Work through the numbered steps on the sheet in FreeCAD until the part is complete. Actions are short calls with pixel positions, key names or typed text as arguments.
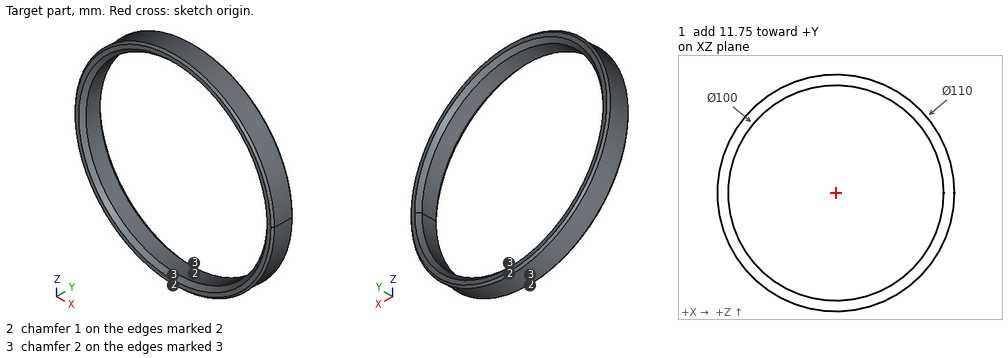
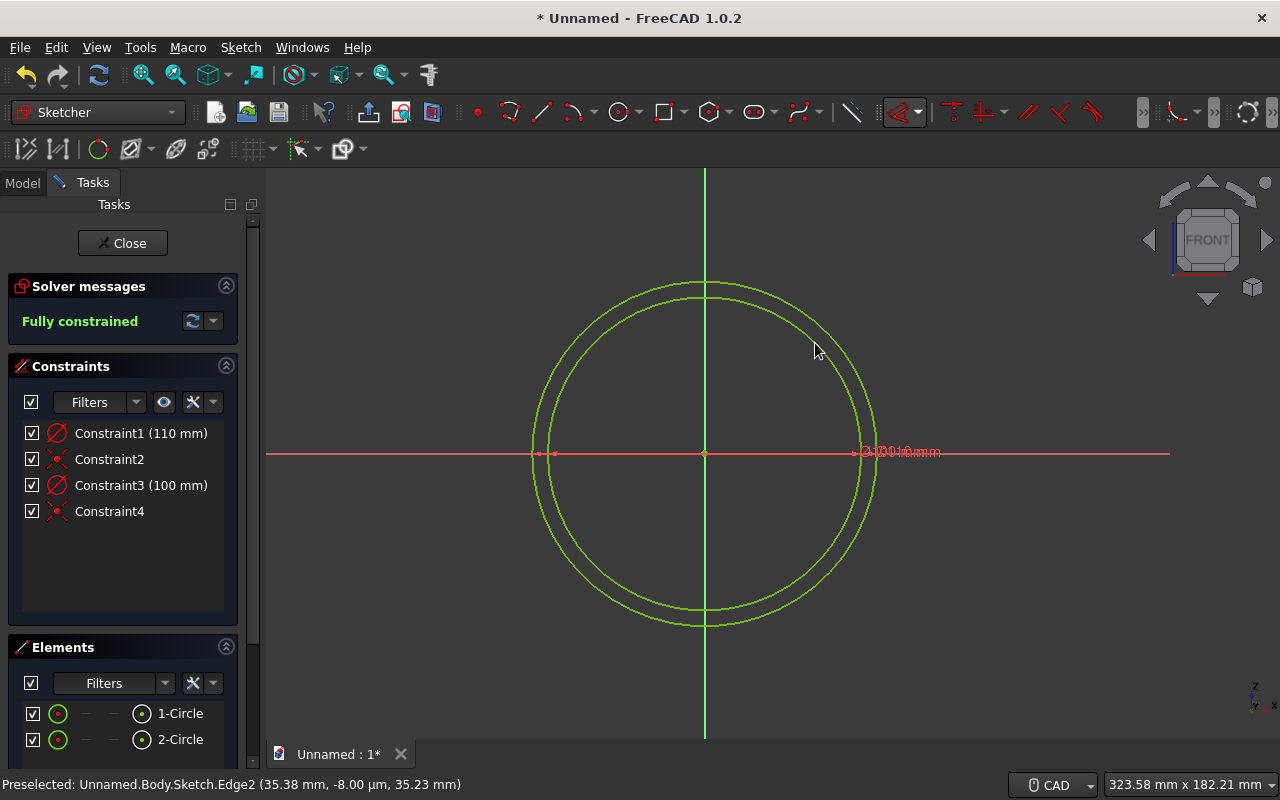
click(123, 243)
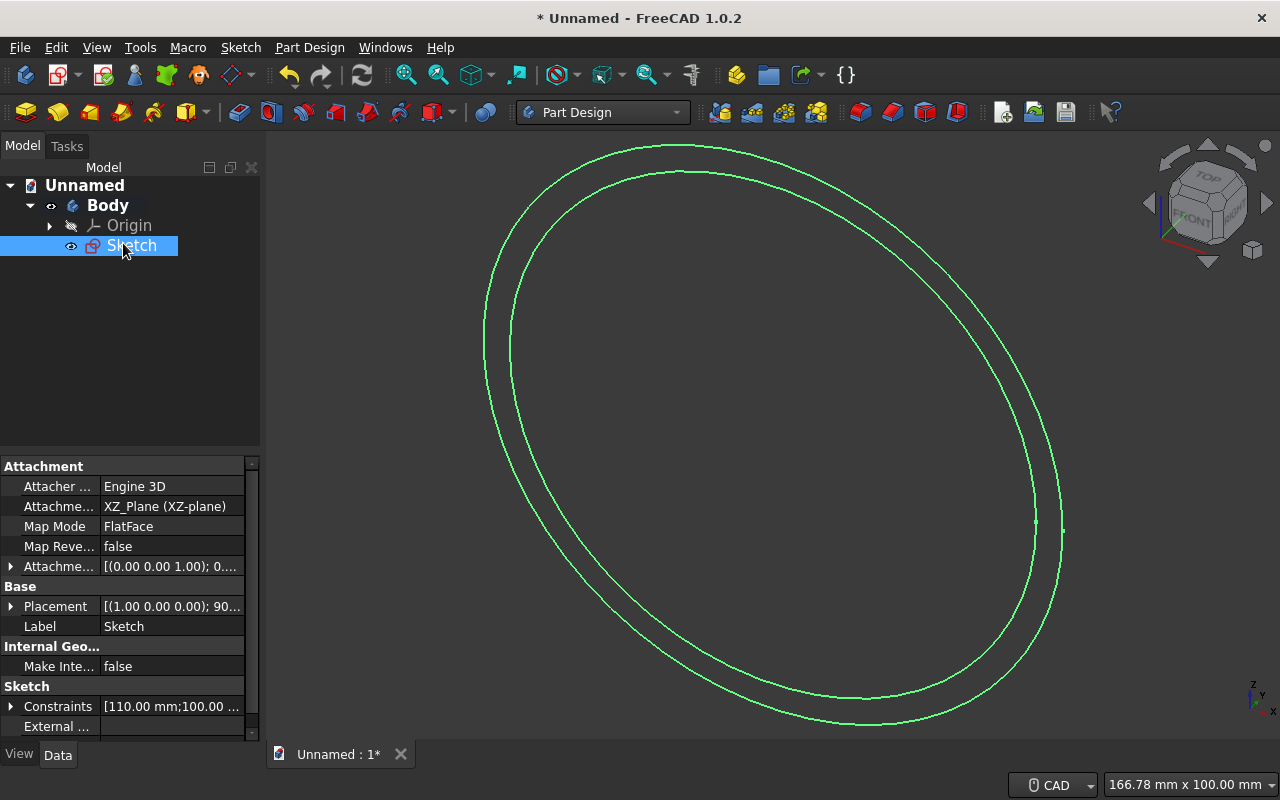
click(26, 112)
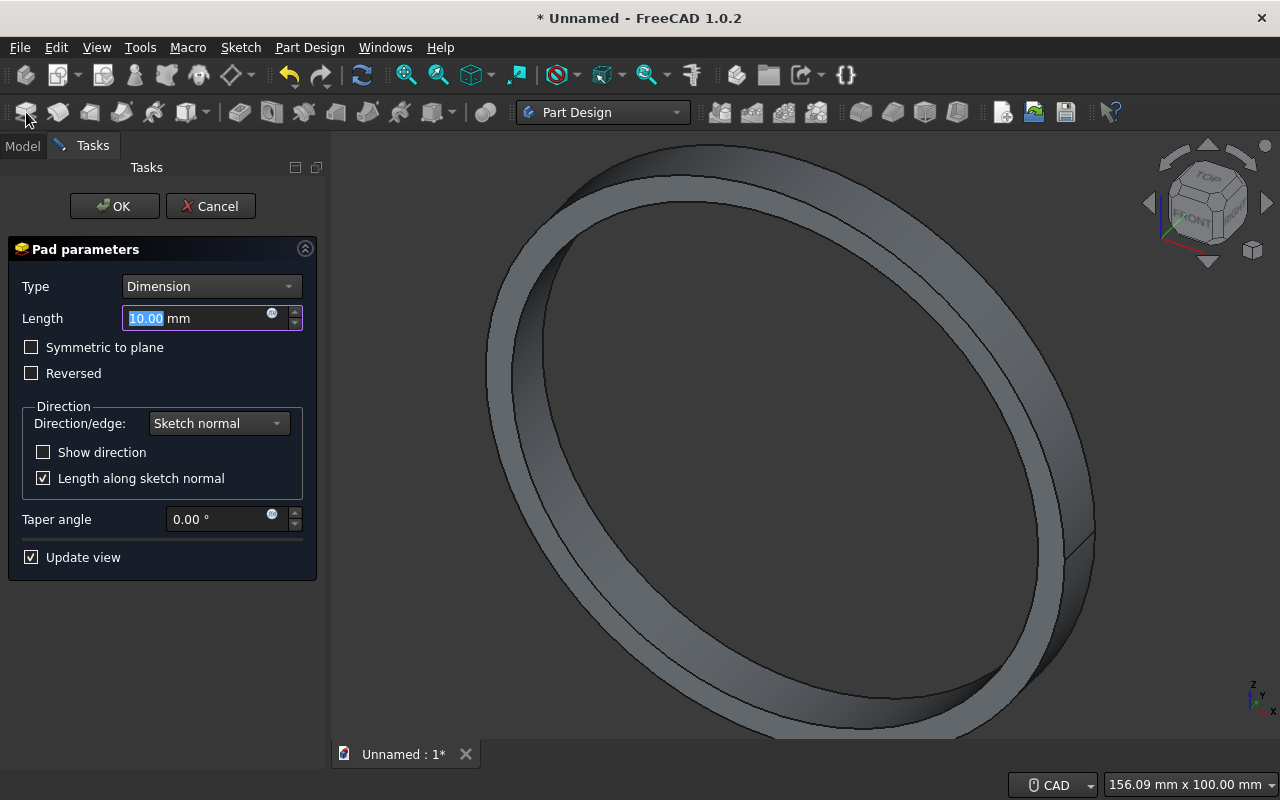
text(11.75)
key(Tab)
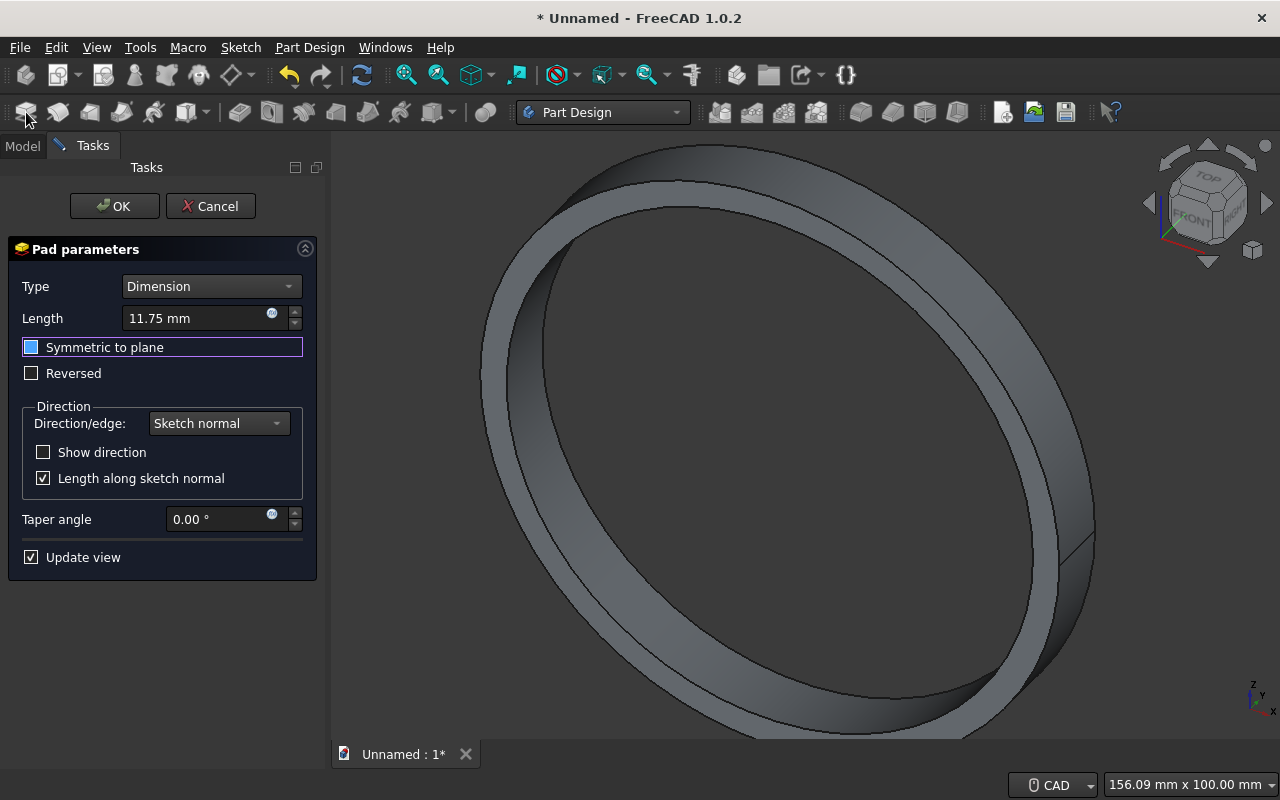
click(30, 373)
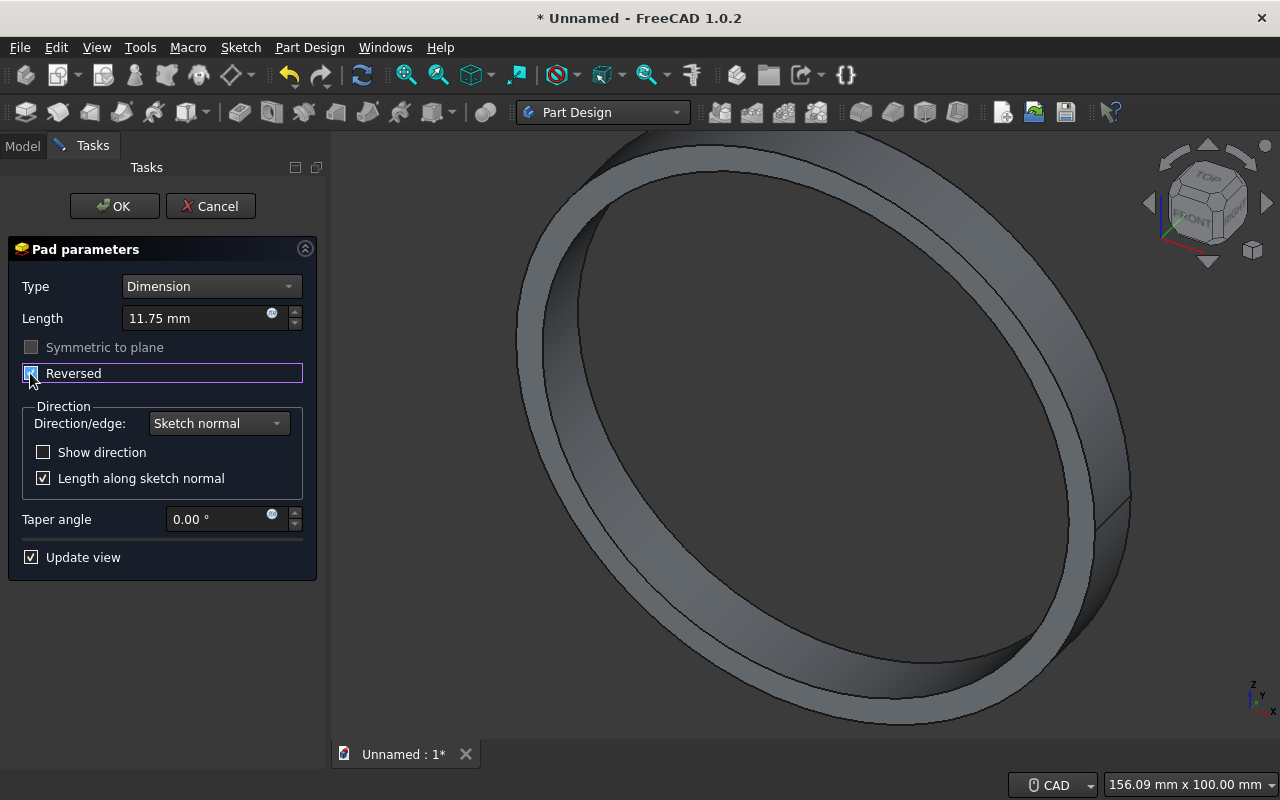
click(115, 206)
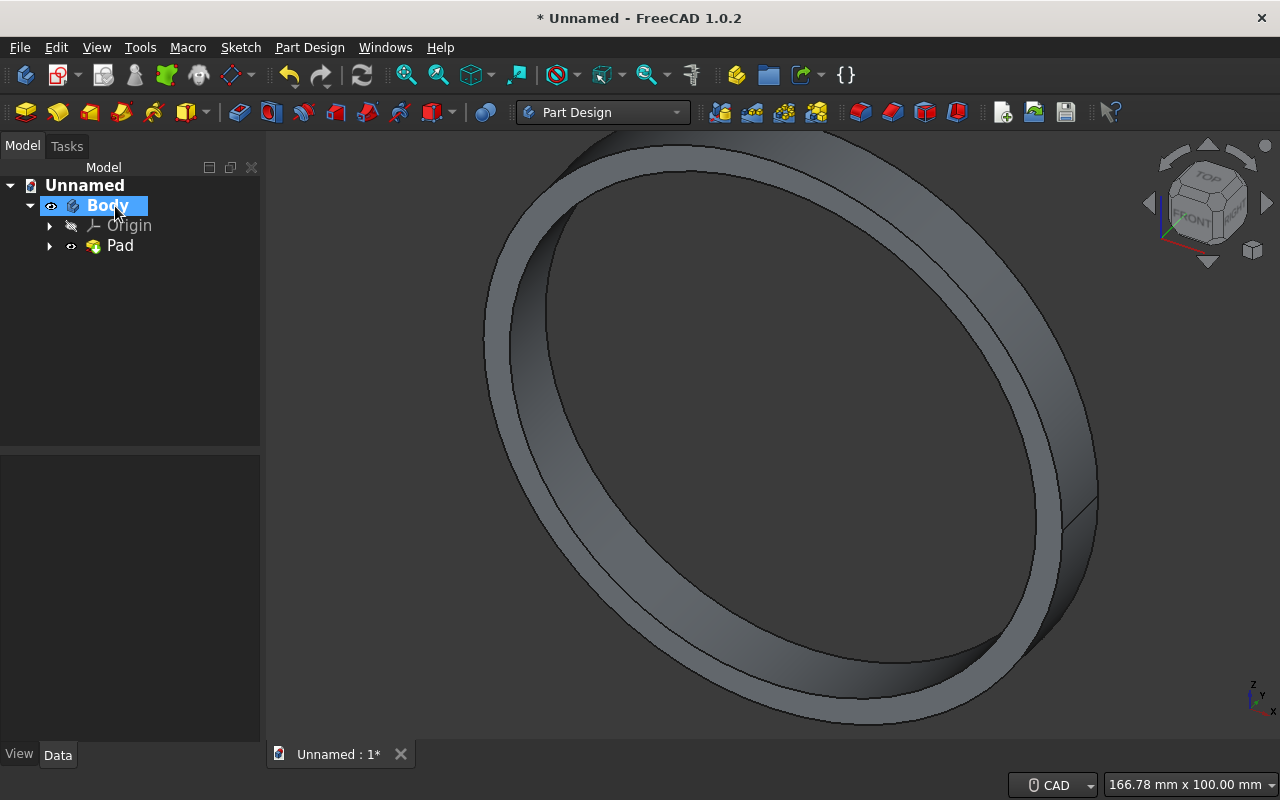
click(408, 76)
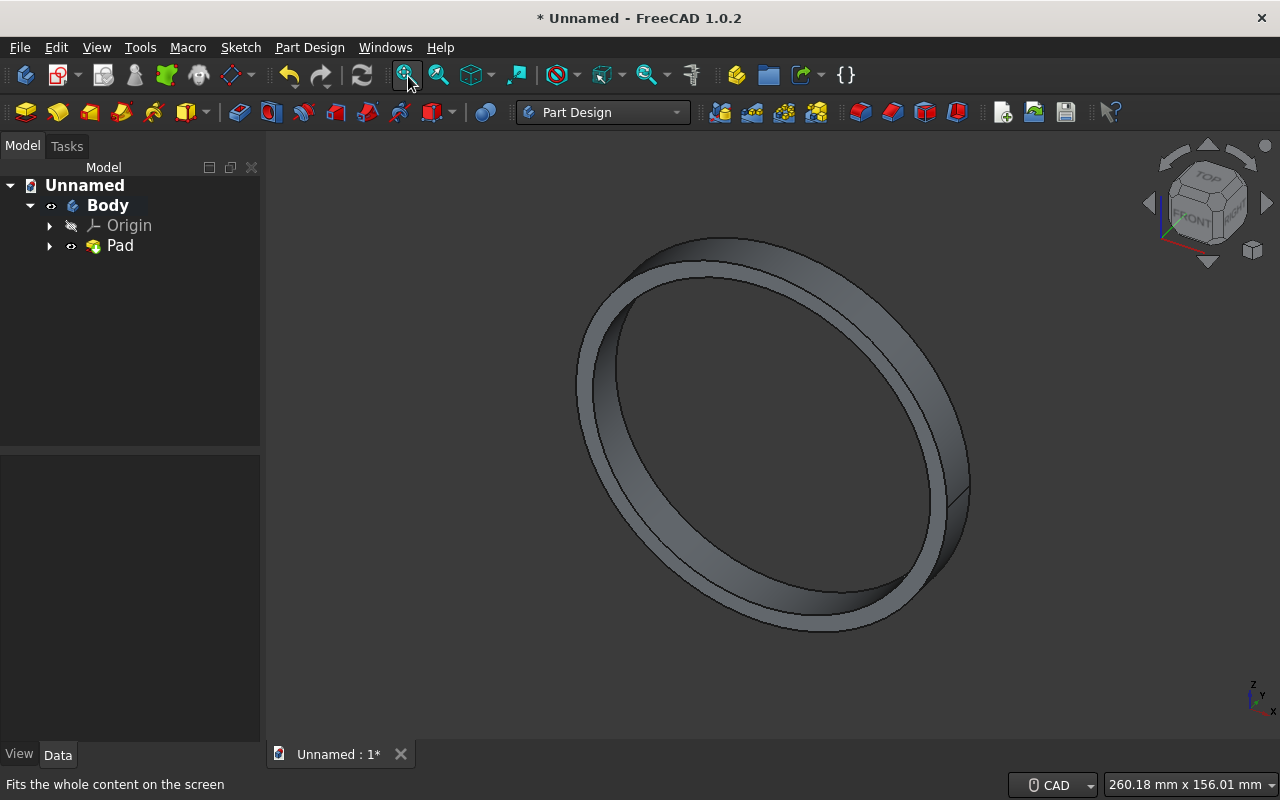
click(611, 292)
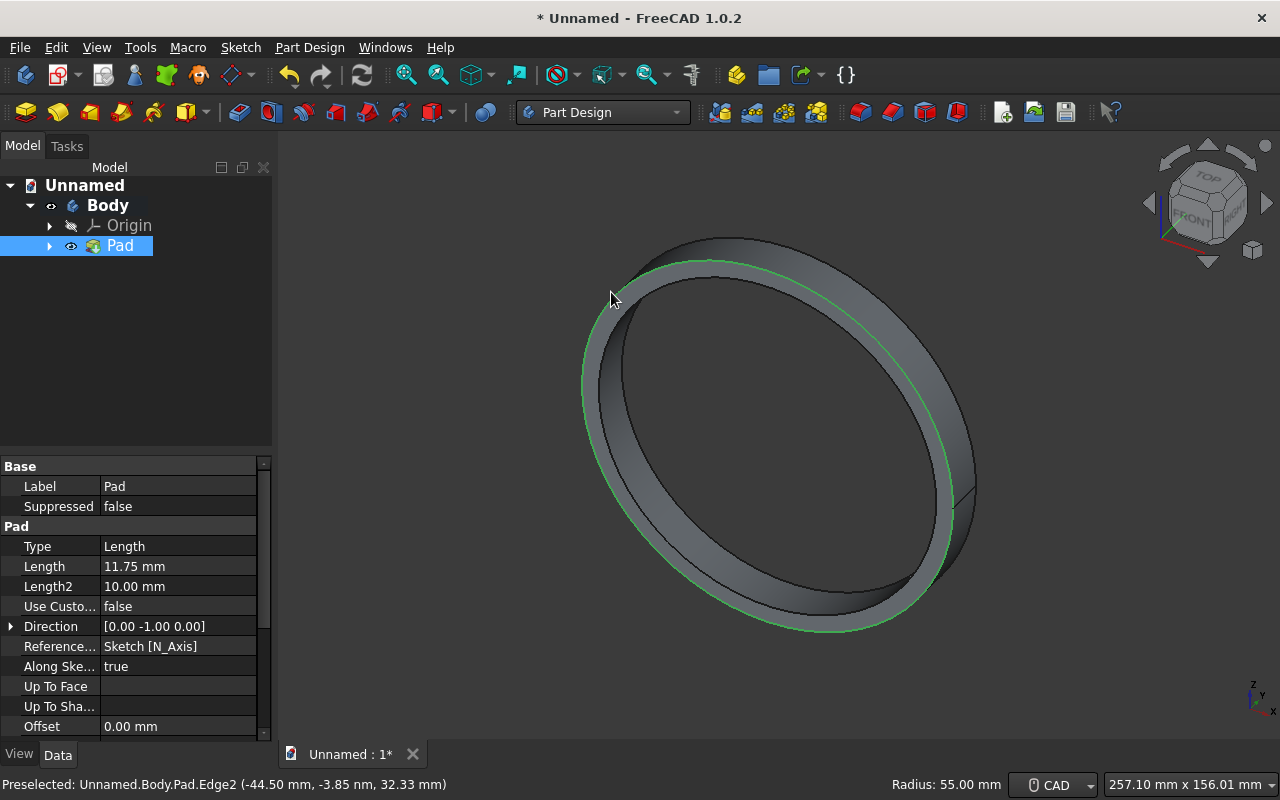
key(0)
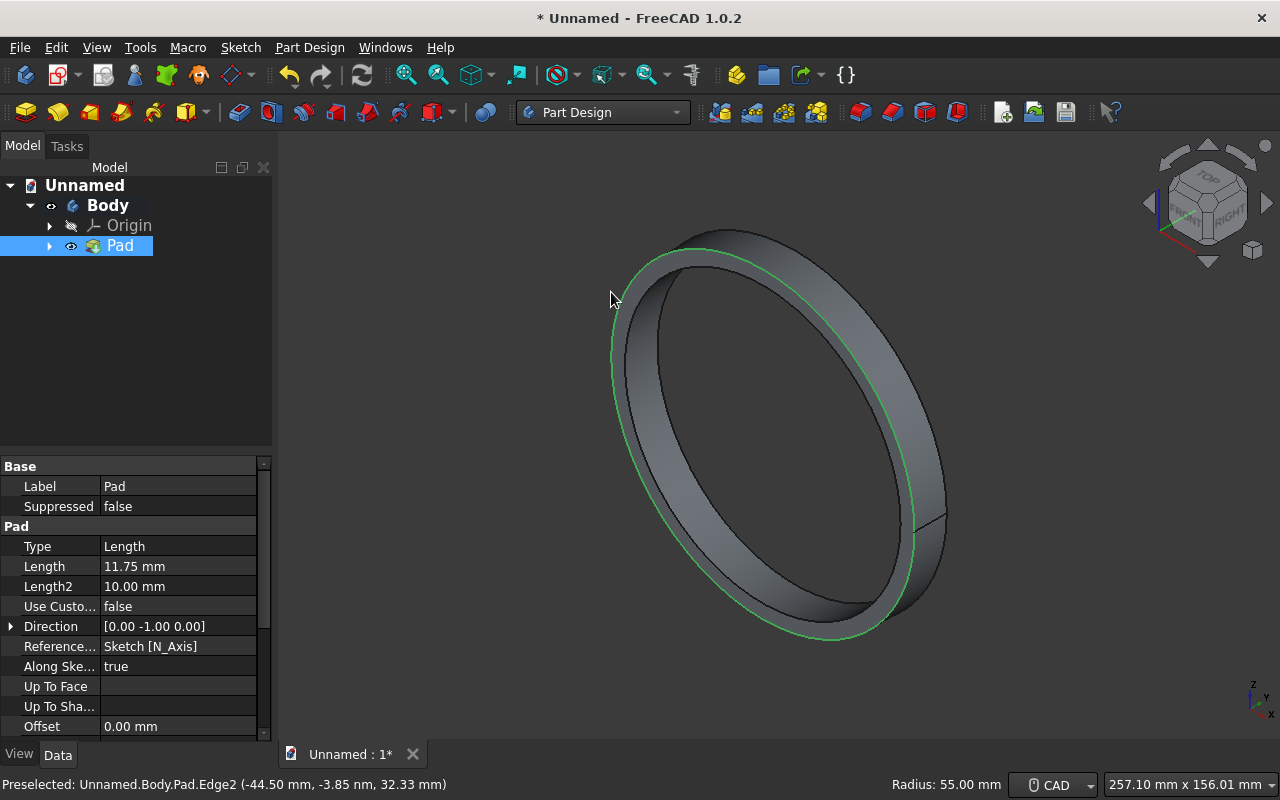
key(2)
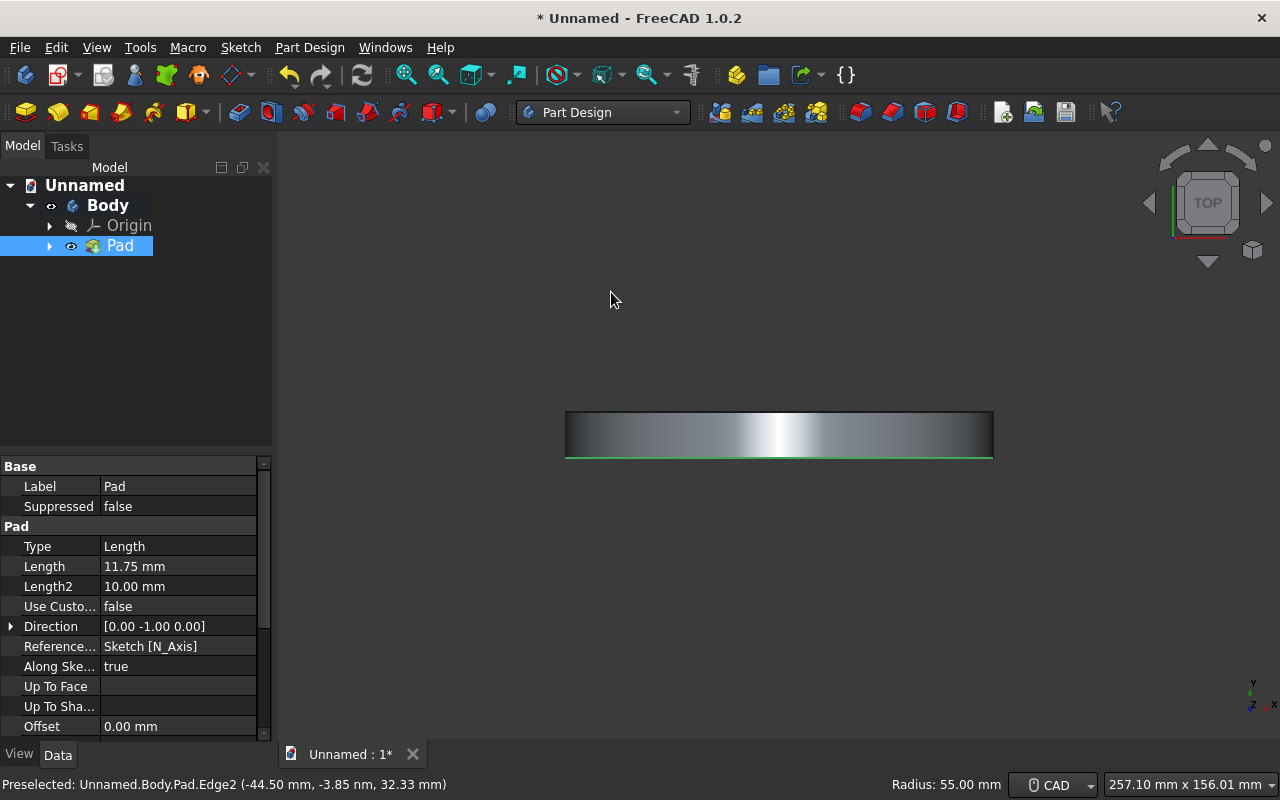
key(v)
key(f)